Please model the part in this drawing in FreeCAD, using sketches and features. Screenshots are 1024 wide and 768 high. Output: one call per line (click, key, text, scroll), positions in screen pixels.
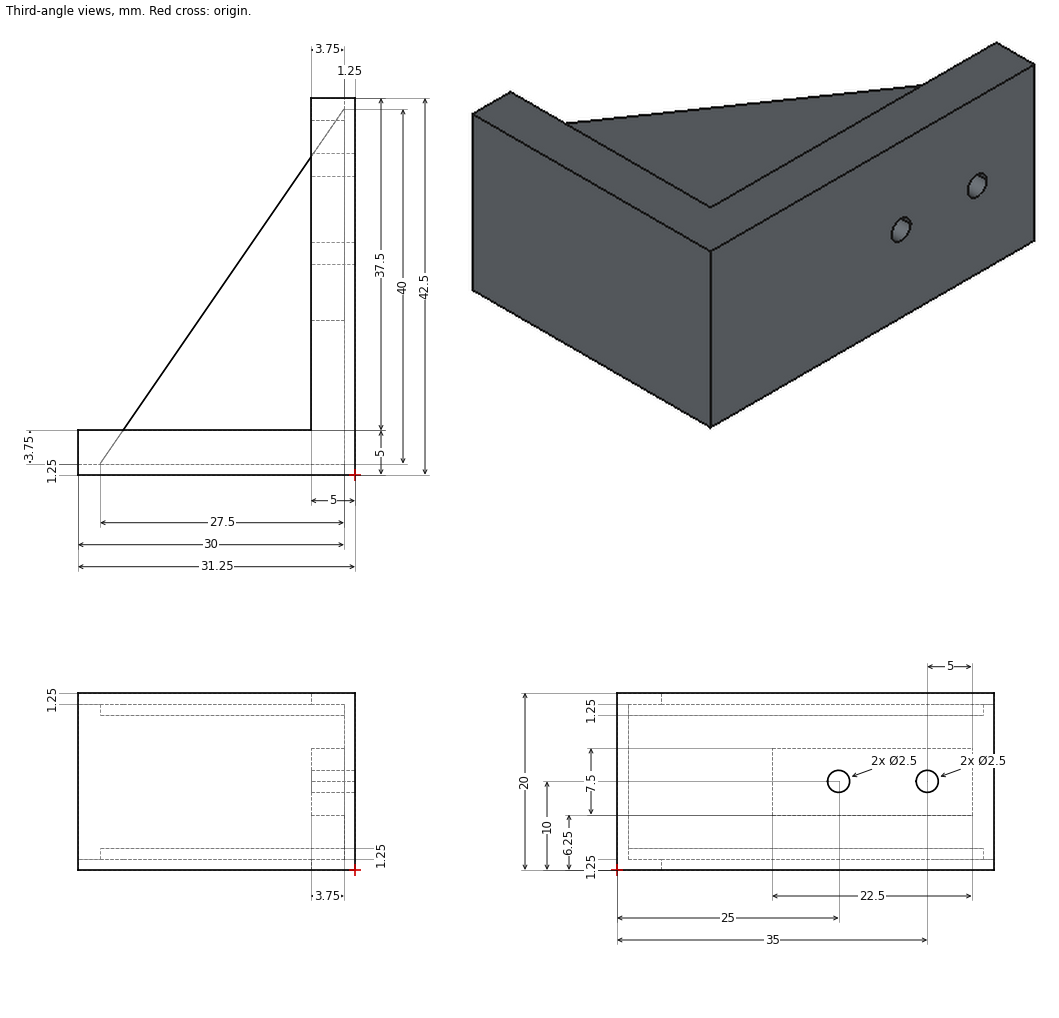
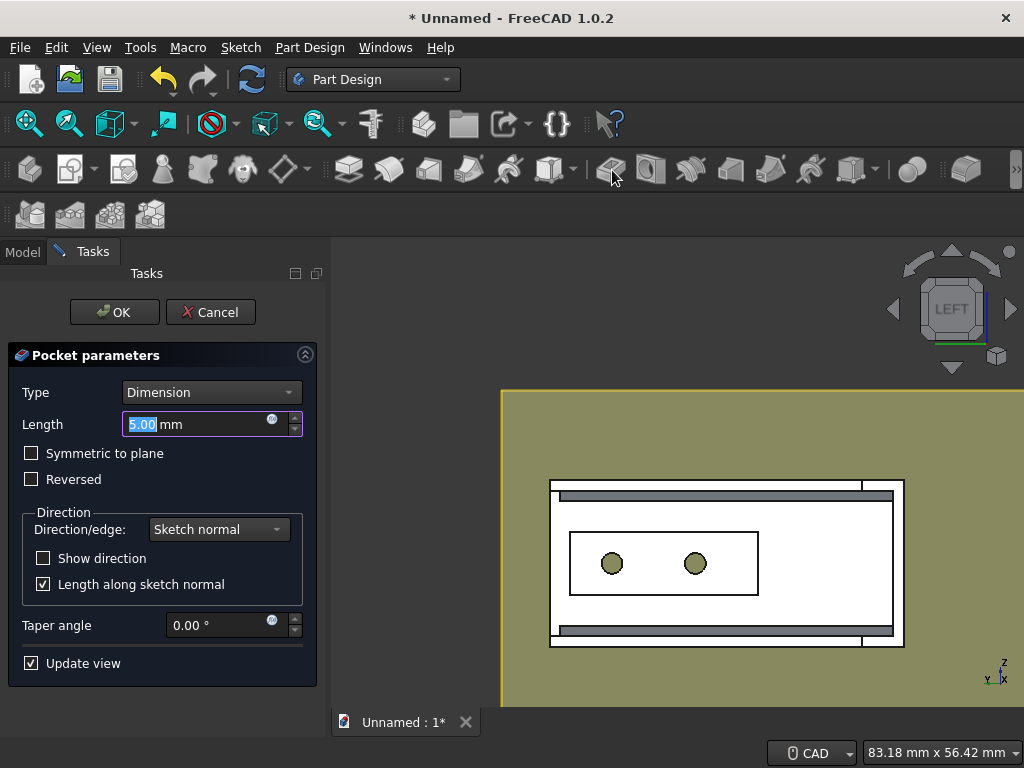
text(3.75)
key(Tab)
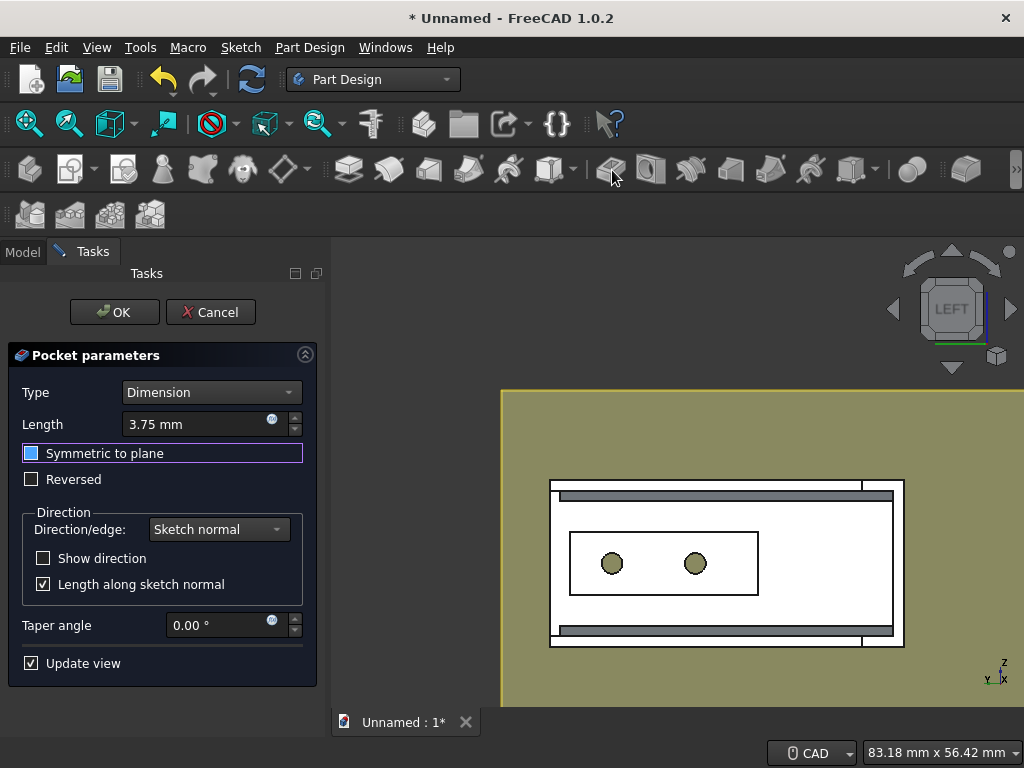
click(115, 312)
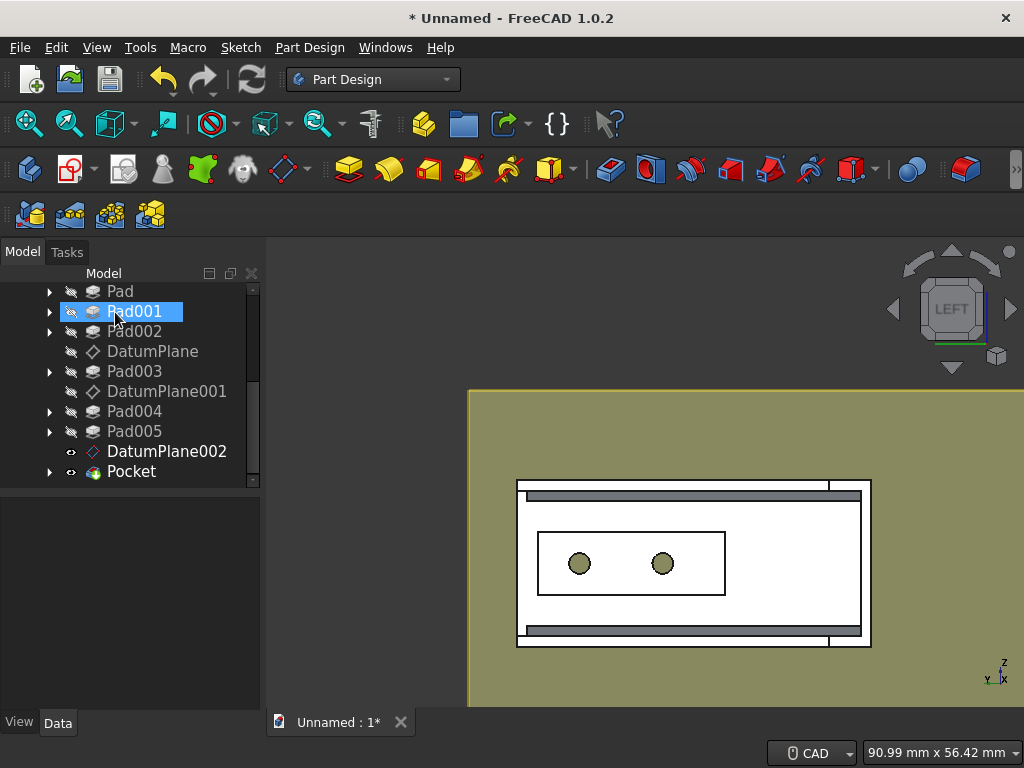
click(116, 452)
key(space)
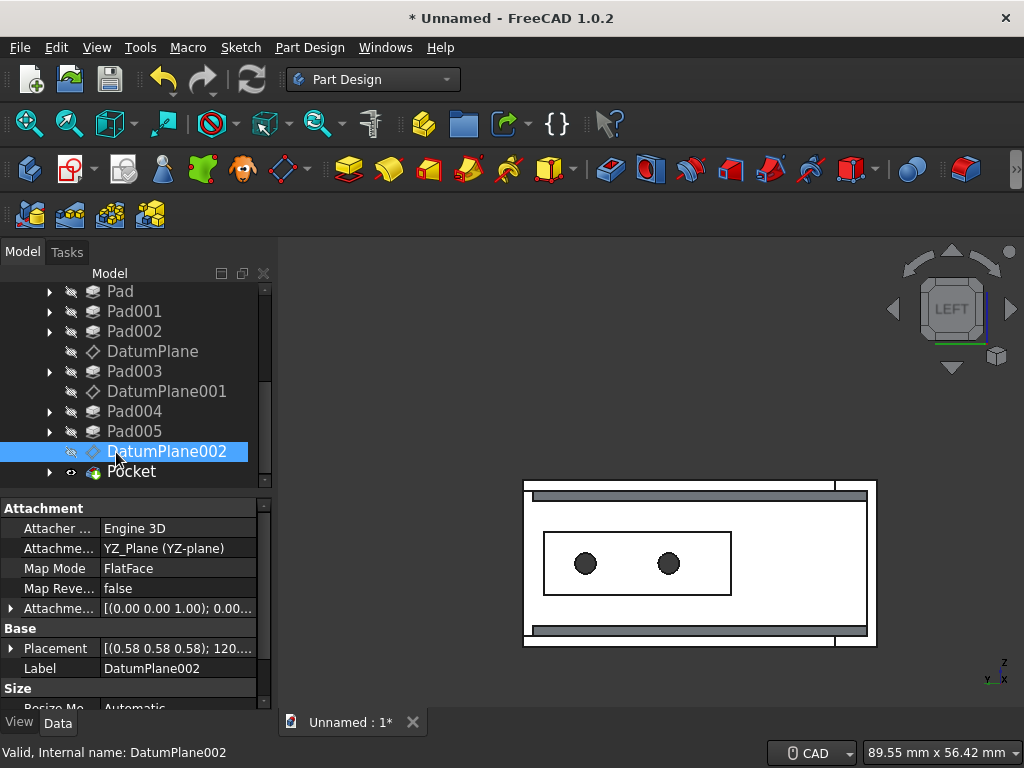
key(0)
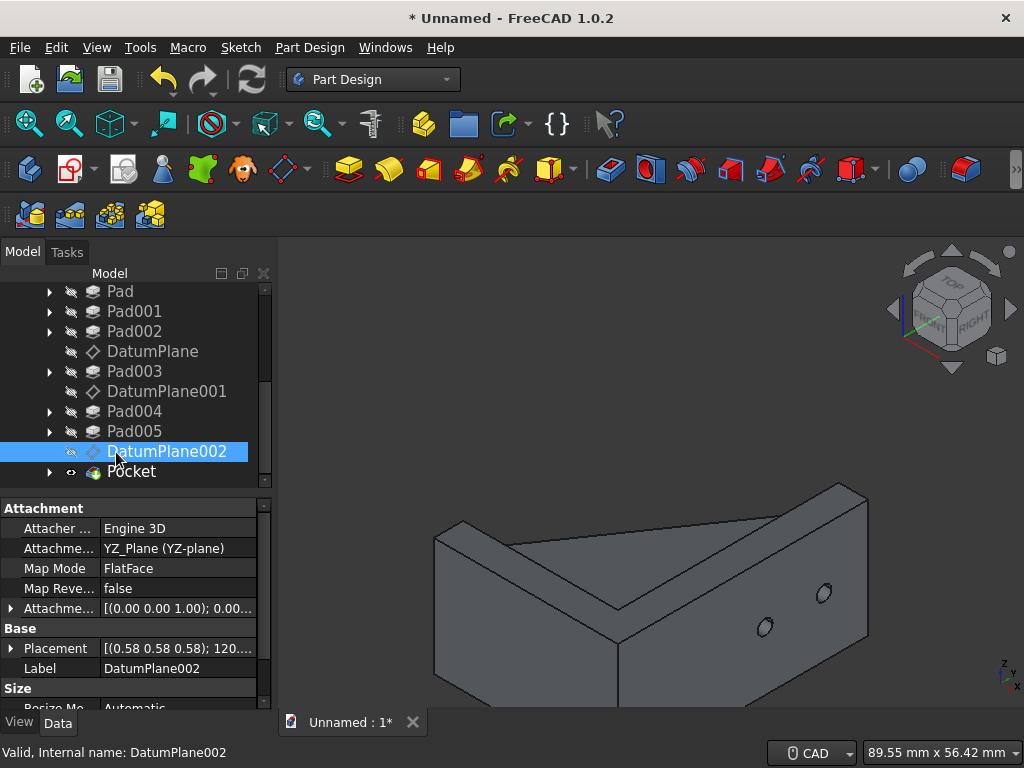
click(30, 124)